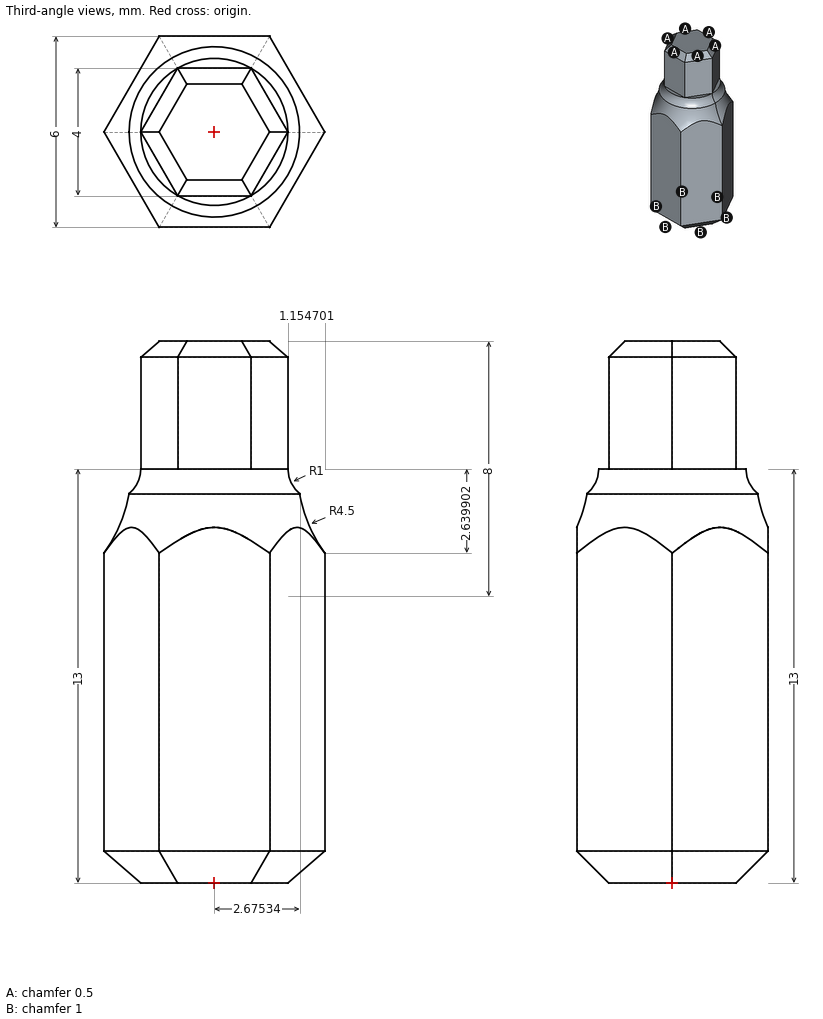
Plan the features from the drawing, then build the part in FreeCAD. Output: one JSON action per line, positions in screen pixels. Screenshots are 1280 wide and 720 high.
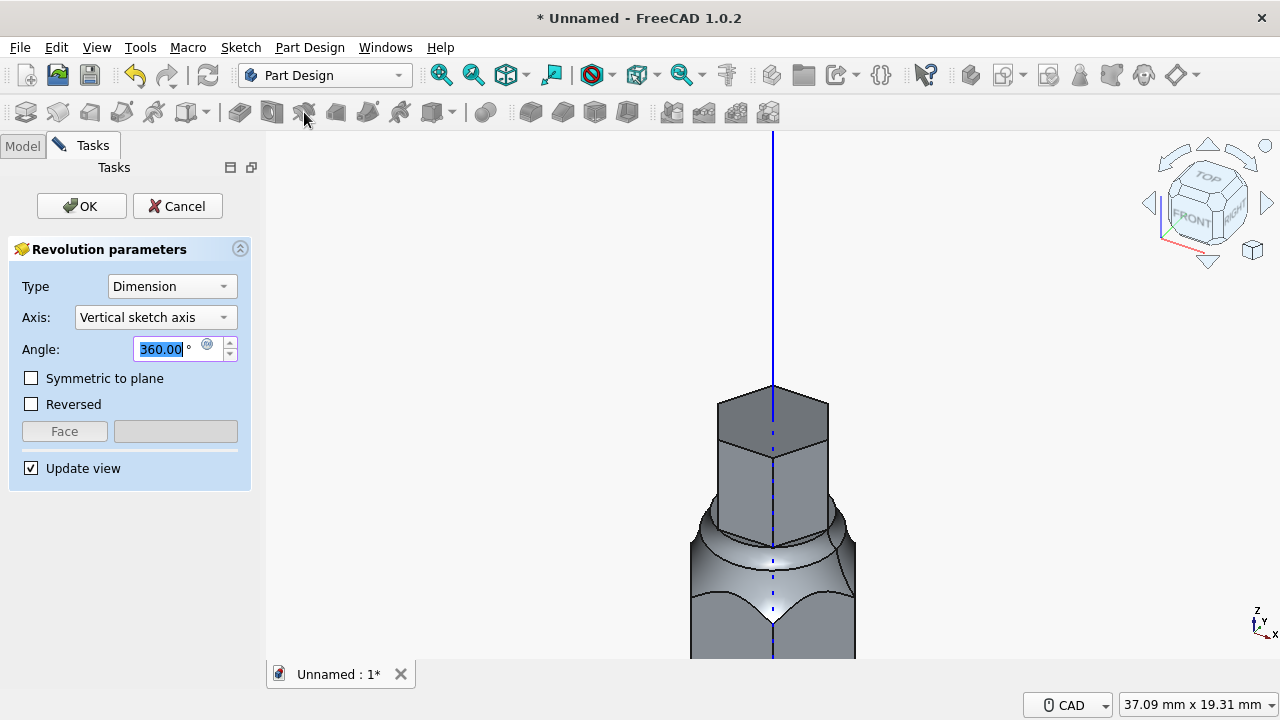
{"action": "left_click", "coordinate": [82, 206]}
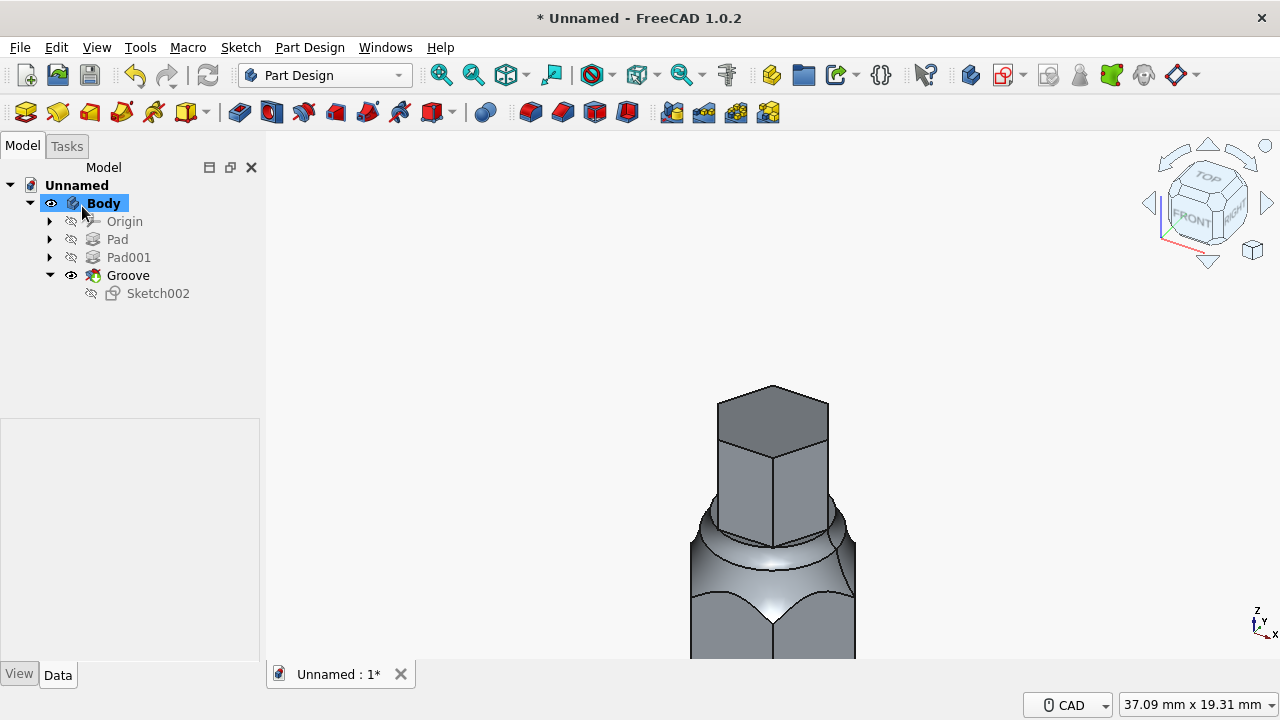
{"action": "left_click", "coordinate": [442, 76]}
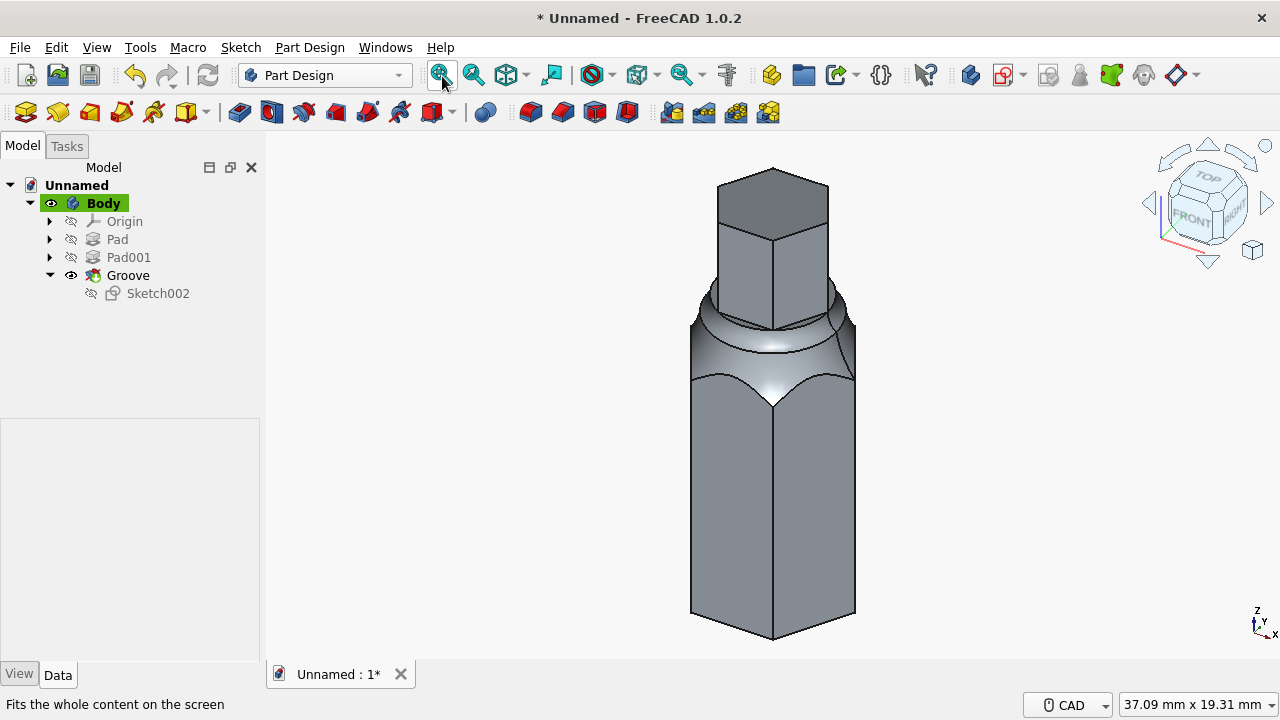
{"action": "left_click", "coordinate": [773, 204]}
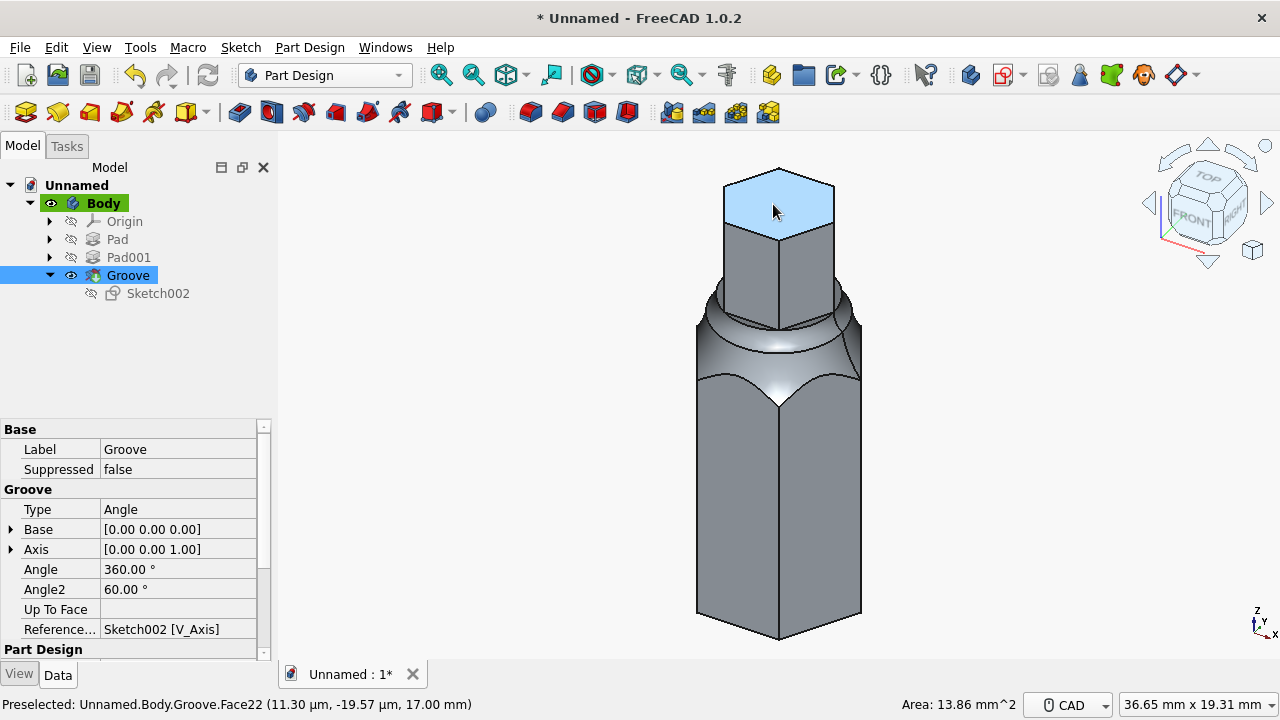
{"action": "left_click", "coordinate": [564, 112]}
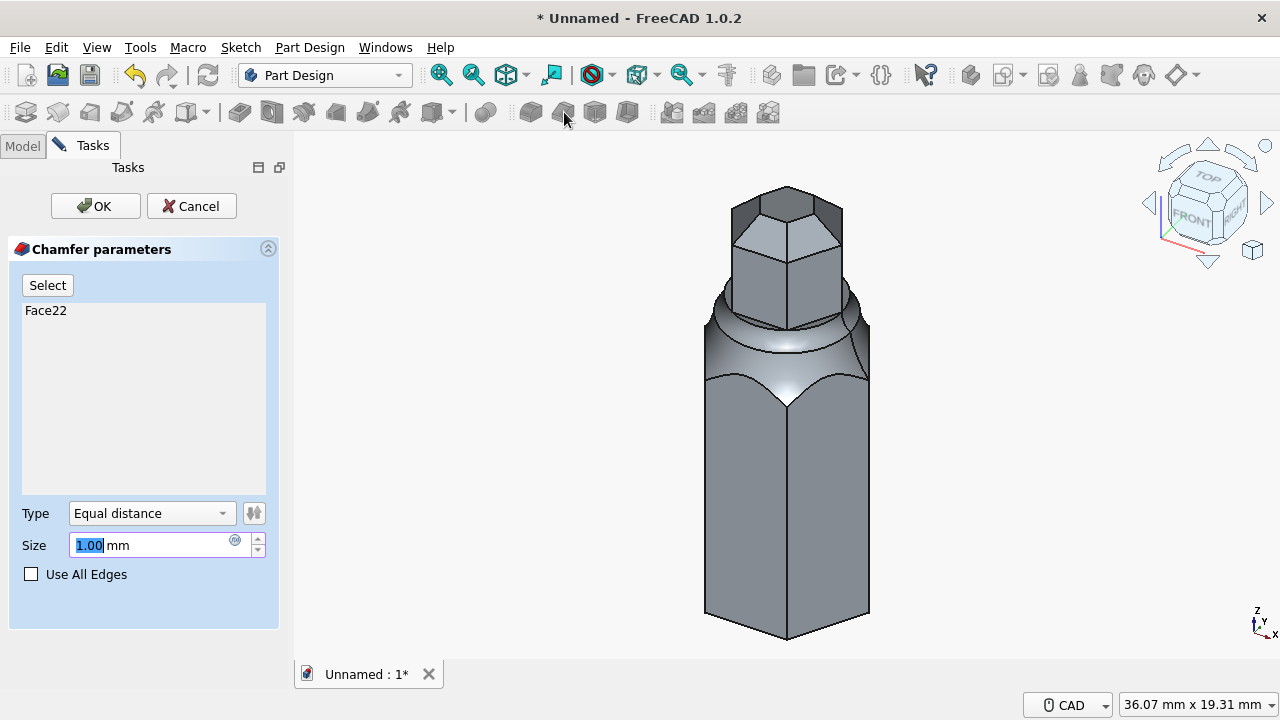
{"action": "type", "text": "0.5"}
{"action": "key", "text": "Tab"}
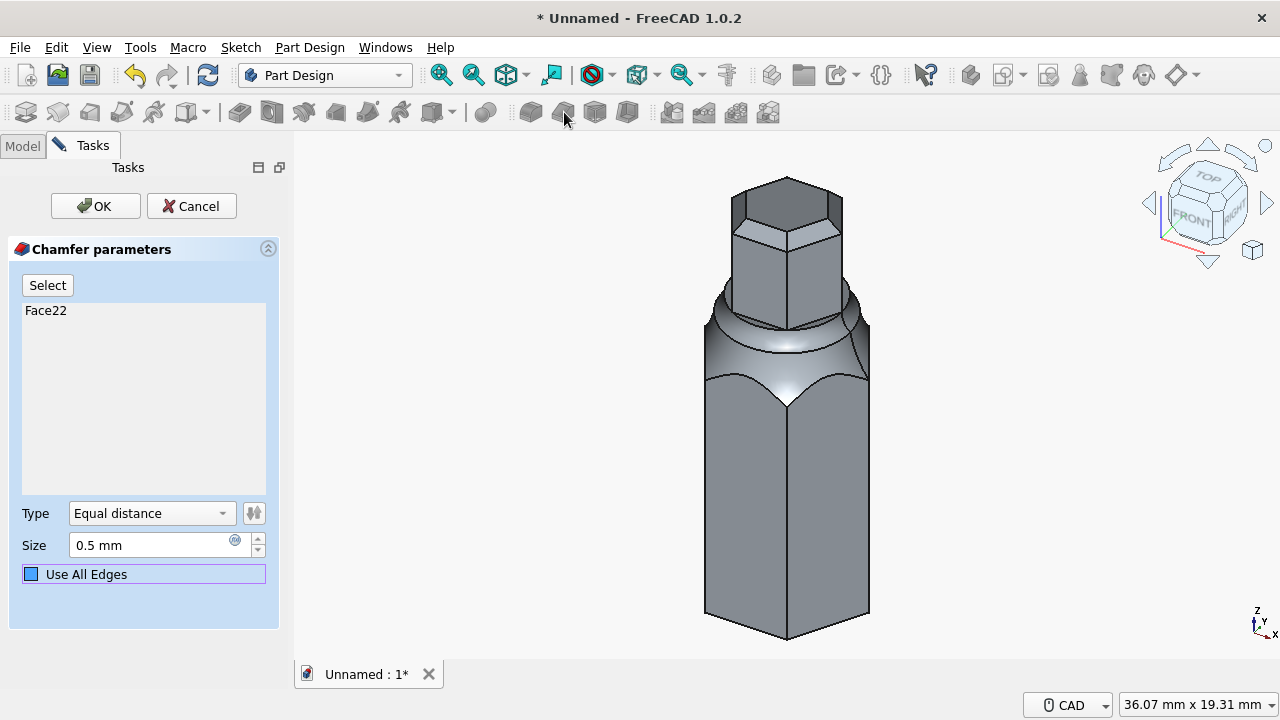
{"action": "left_click", "coordinate": [96, 206]}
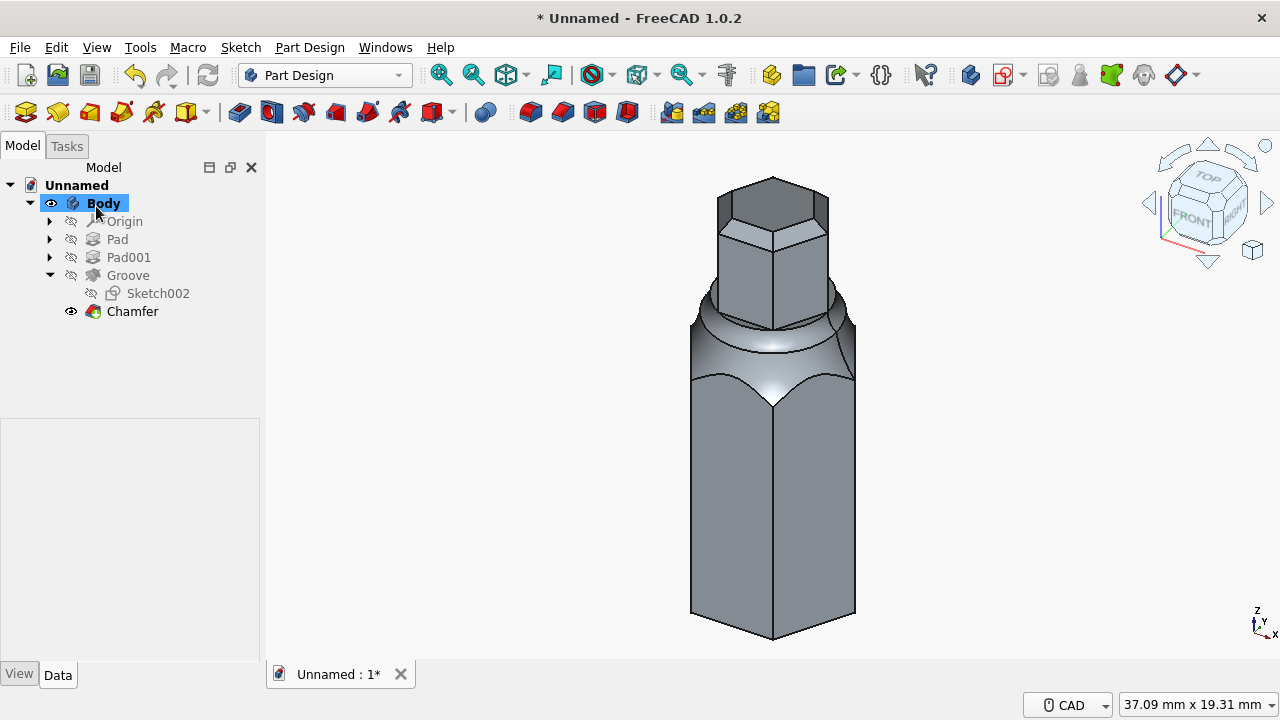
{"action": "key", "text": "0"}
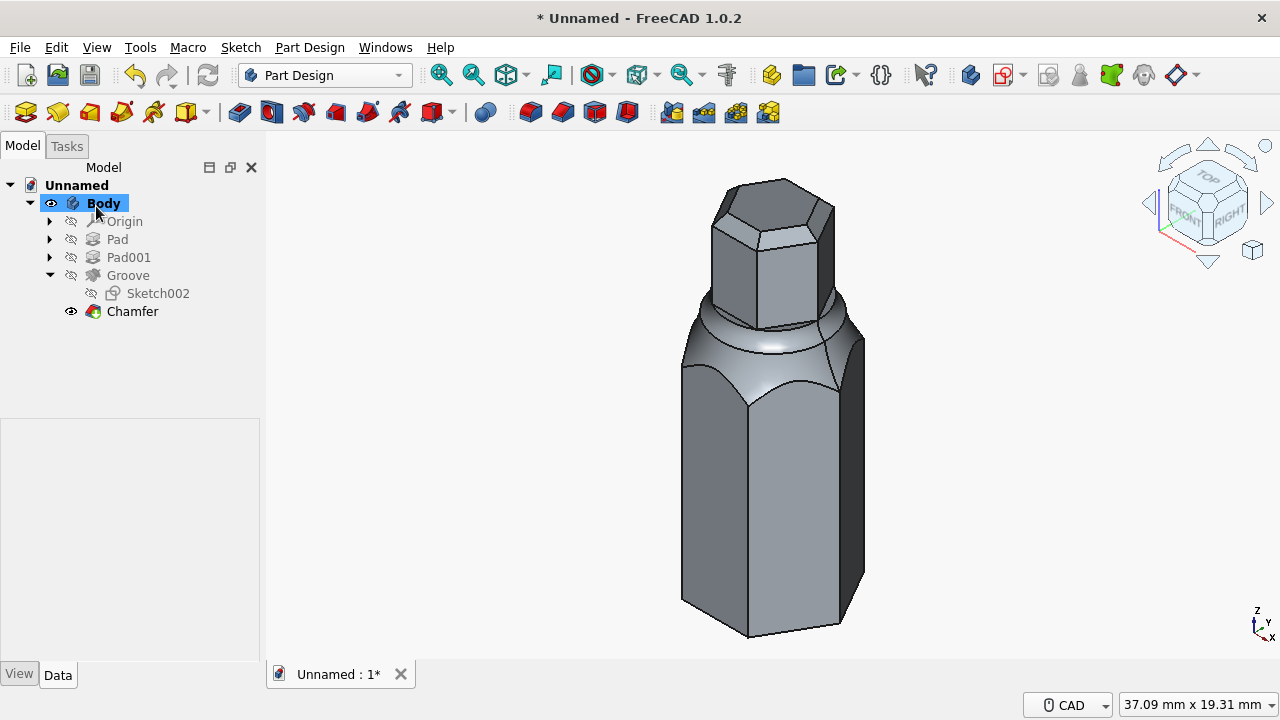
{"action": "key", "text": "2"}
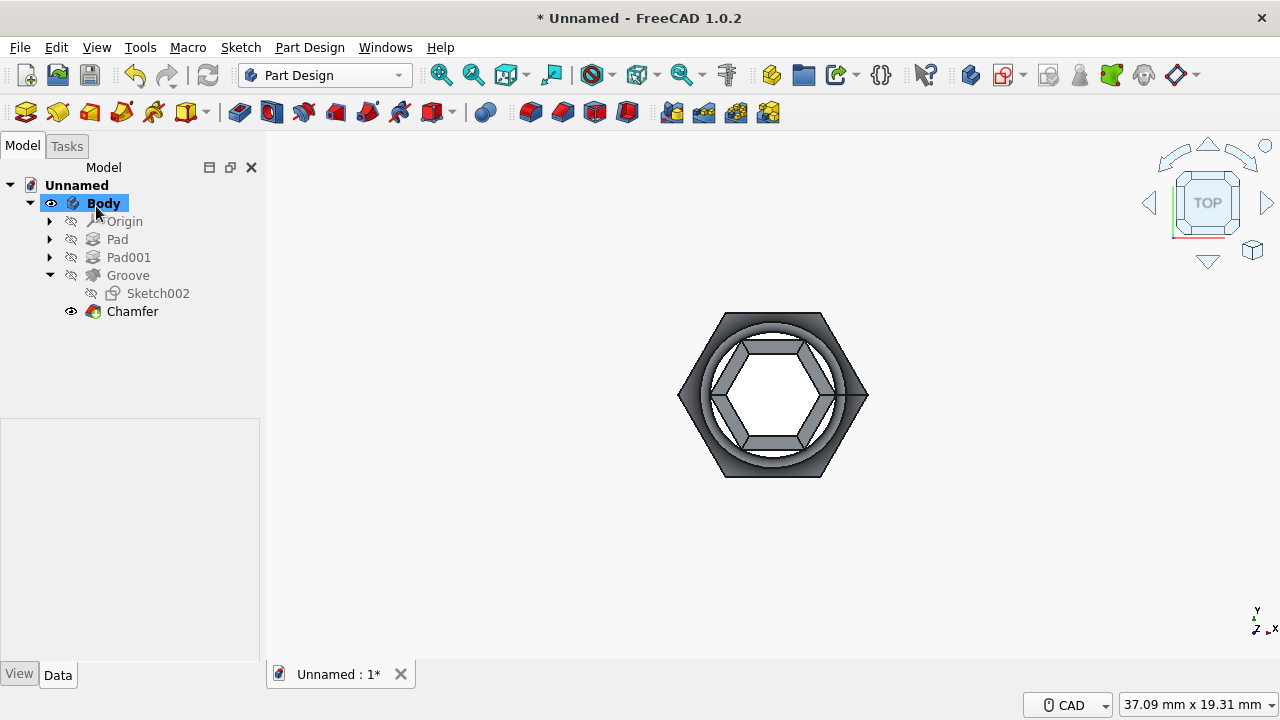
{"action": "left_click", "coordinate": [442, 76]}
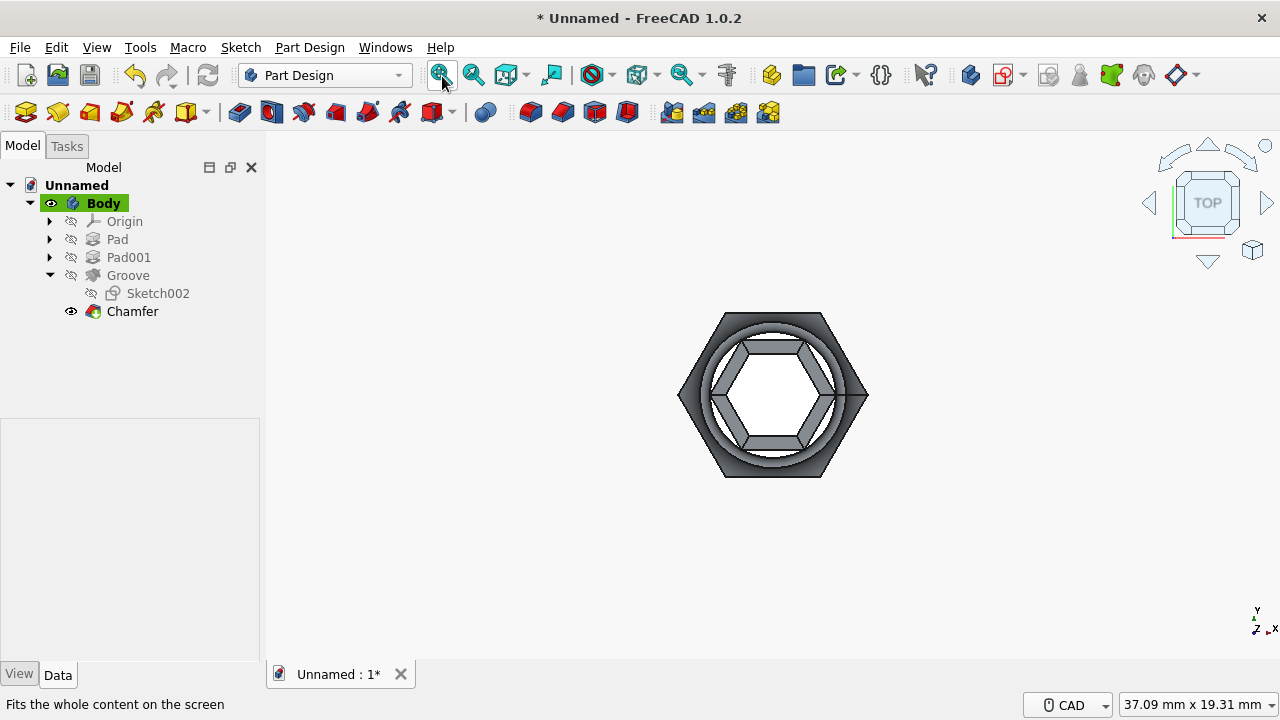
{"action": "key", "text": "1"}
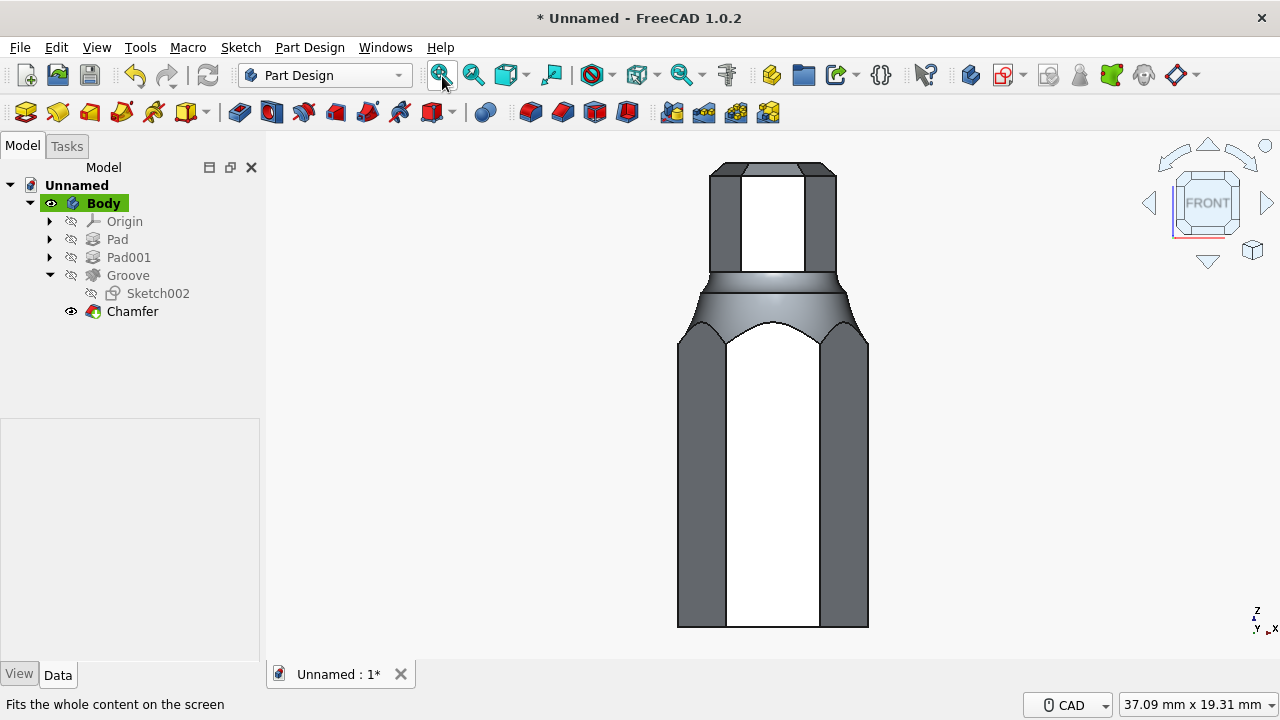
{"action": "key", "text": "3"}